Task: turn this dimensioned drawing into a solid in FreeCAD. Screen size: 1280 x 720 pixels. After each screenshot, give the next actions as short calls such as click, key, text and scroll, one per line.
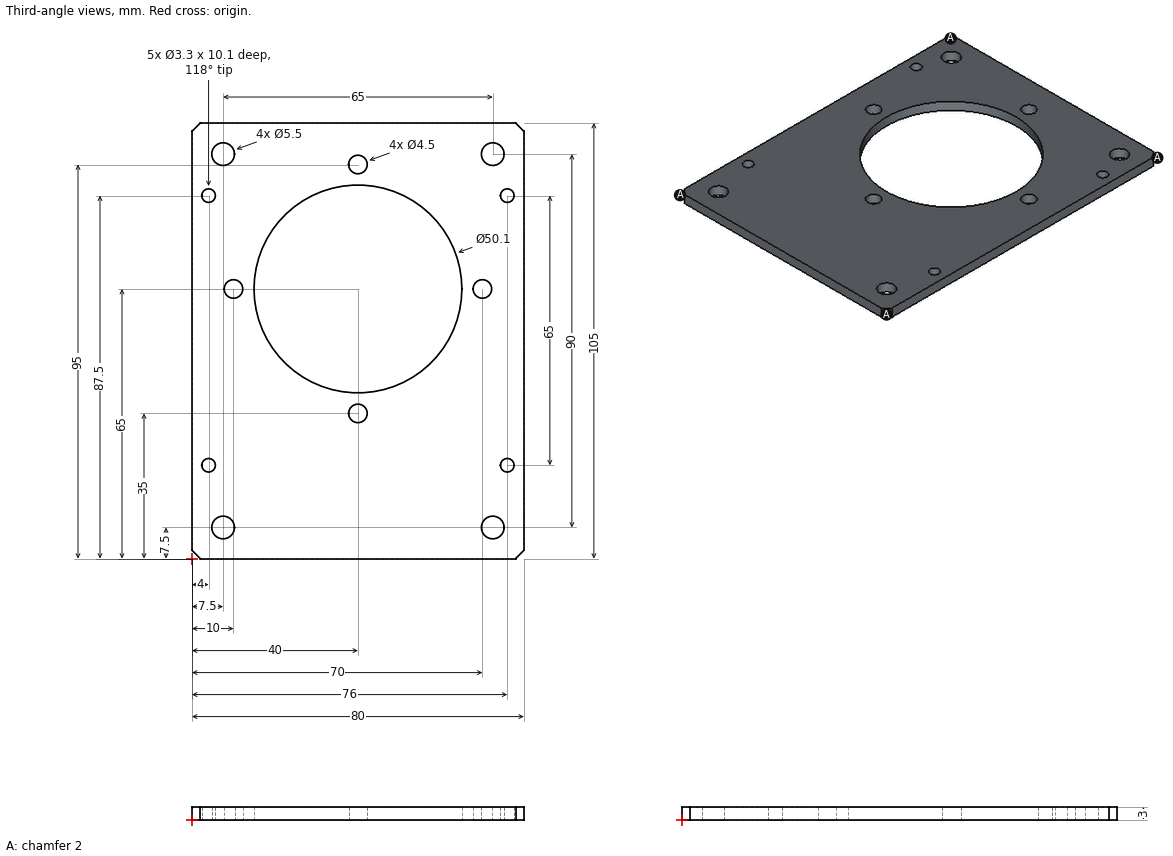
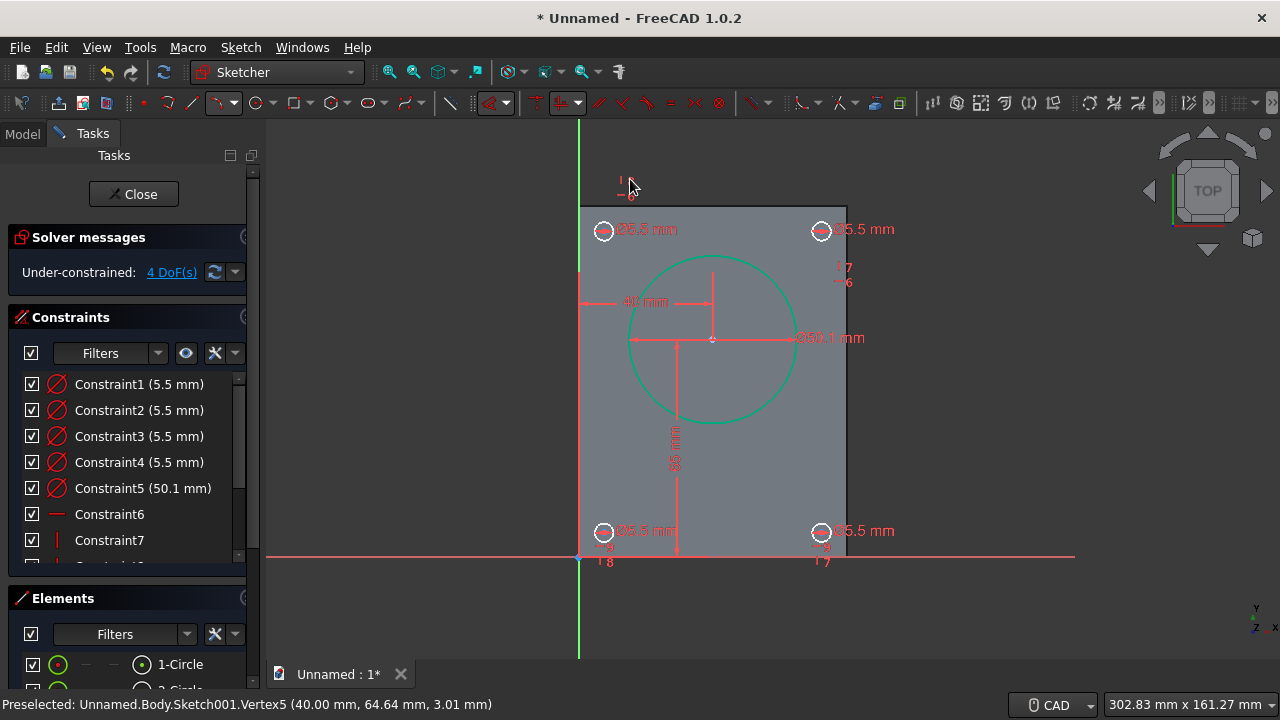
scroll(604, 231, up, 3)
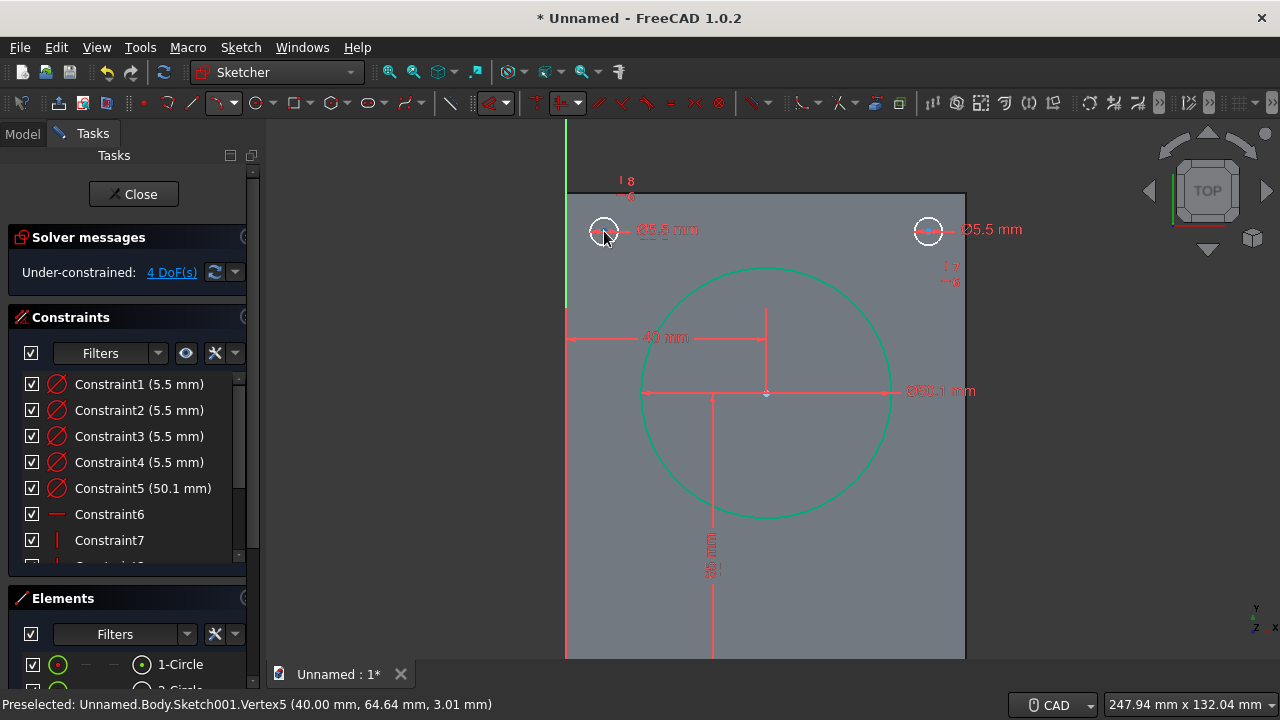
click(604, 232)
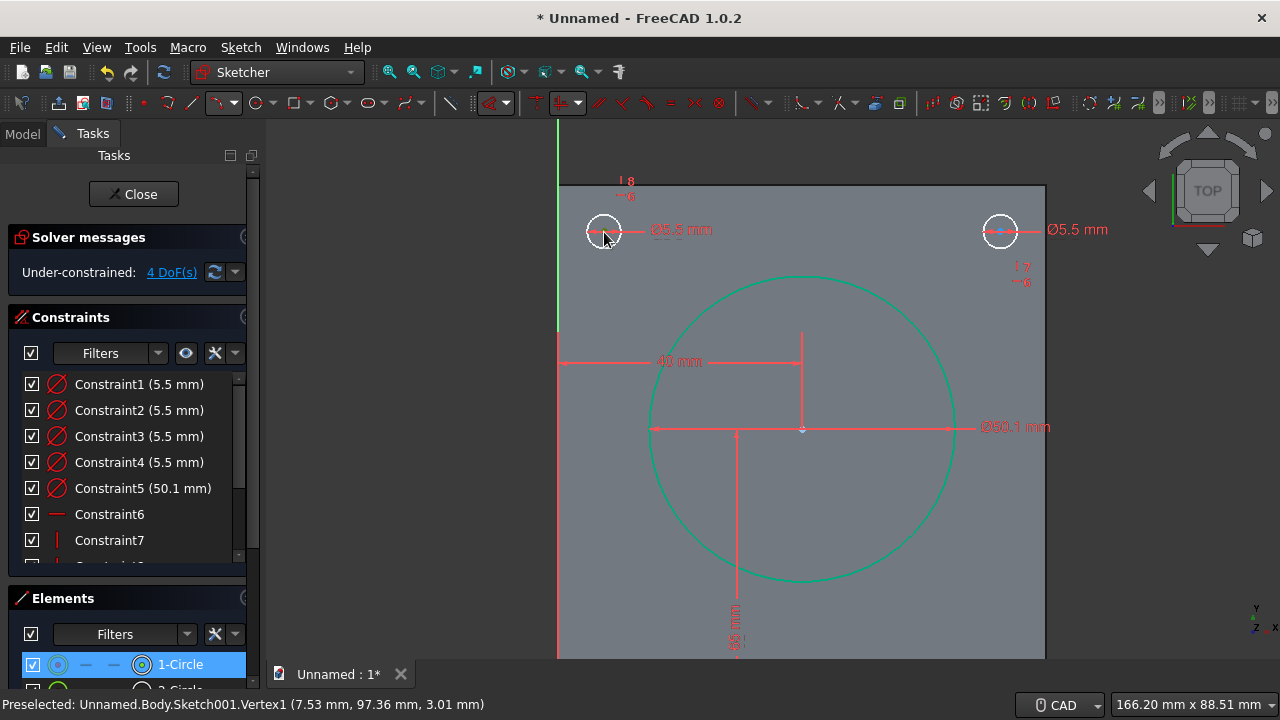
click(508, 104)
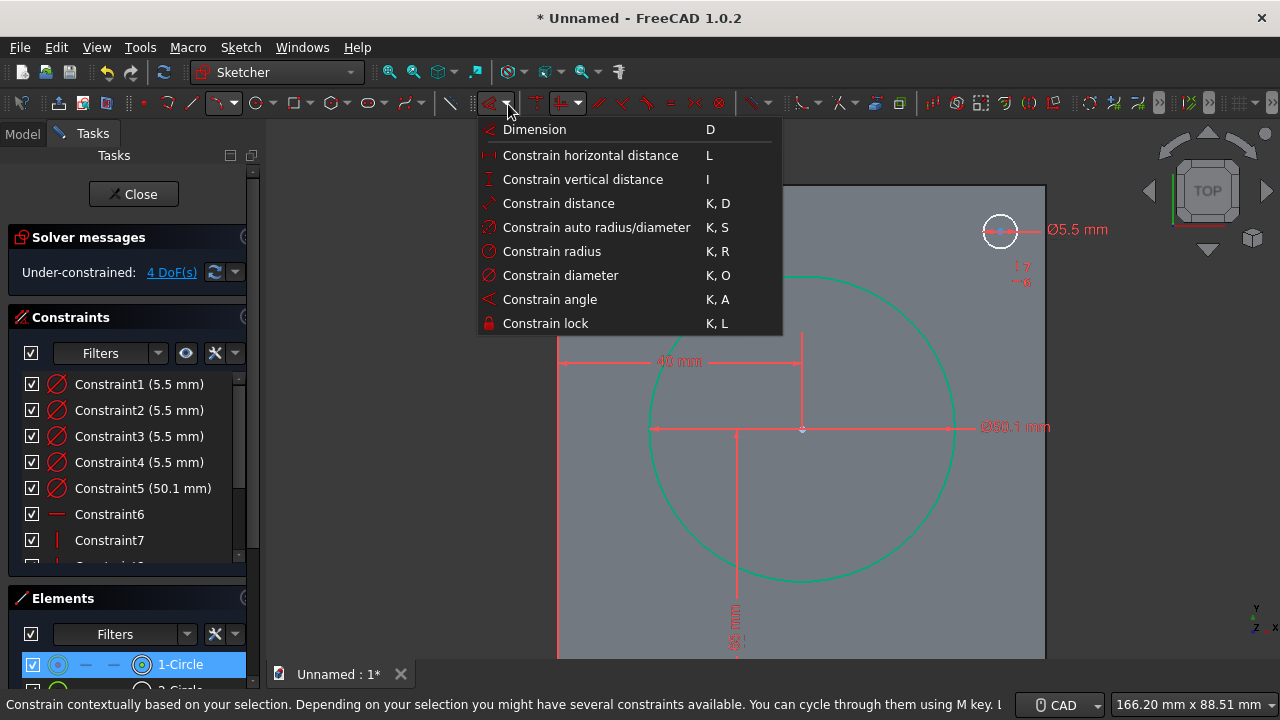
click(630, 155)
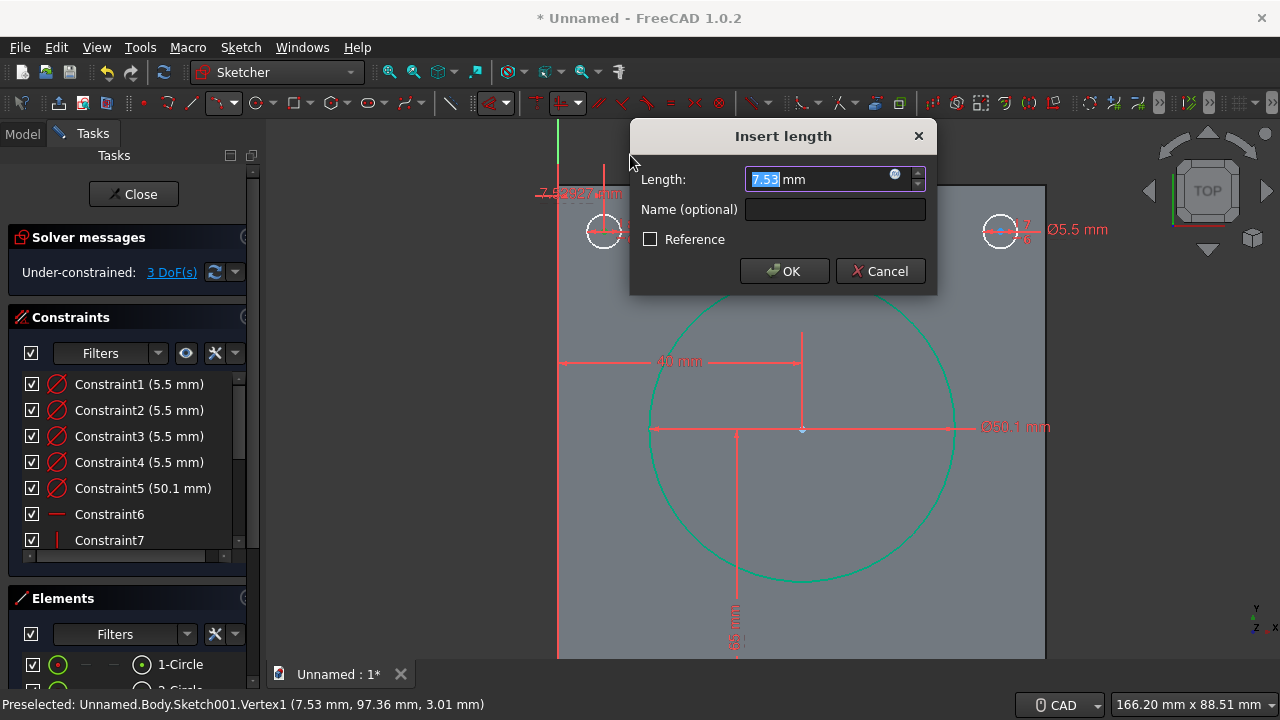
text(7.5)
key(Return)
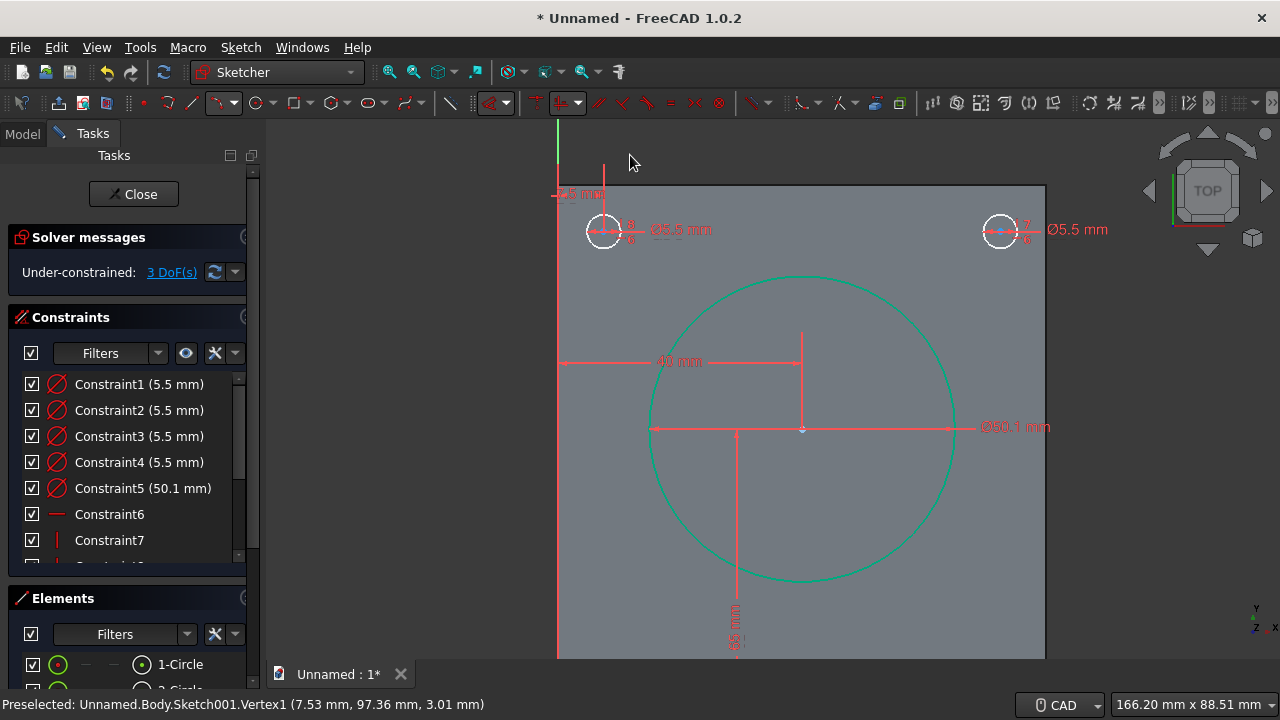
scroll(603, 230, down, 3)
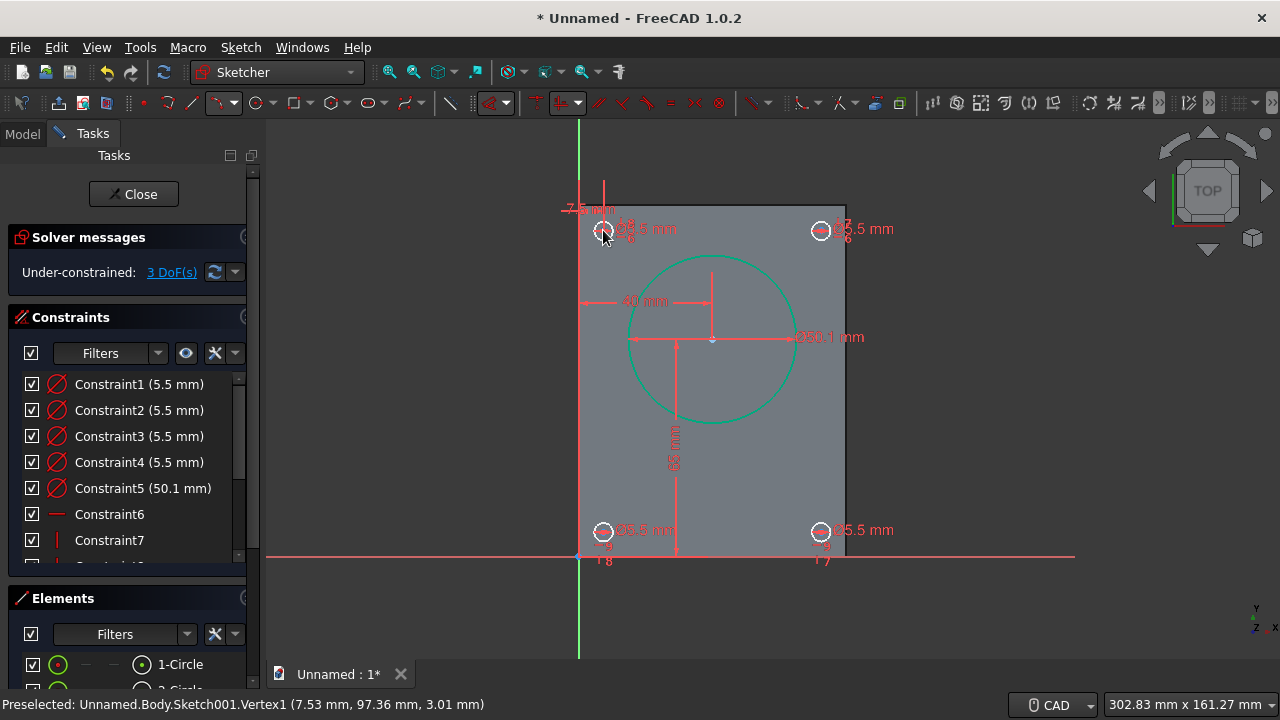
scroll(821, 532, up, 3)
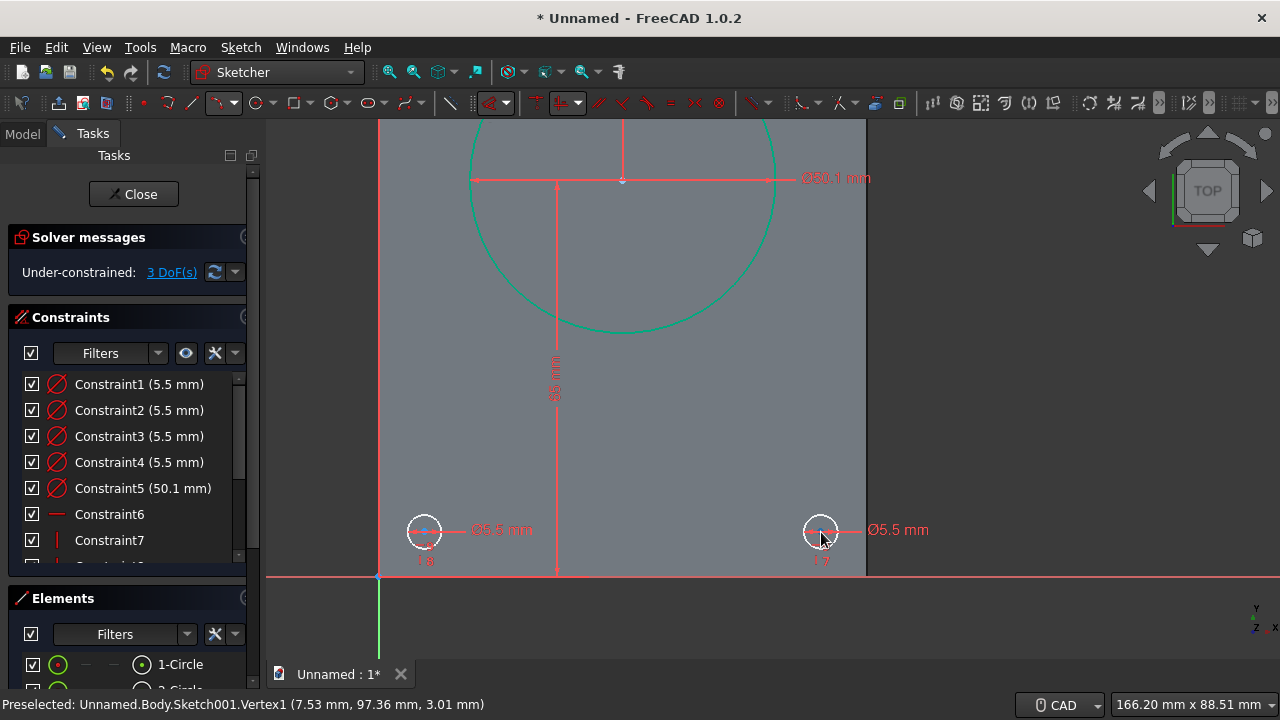
click(821, 532)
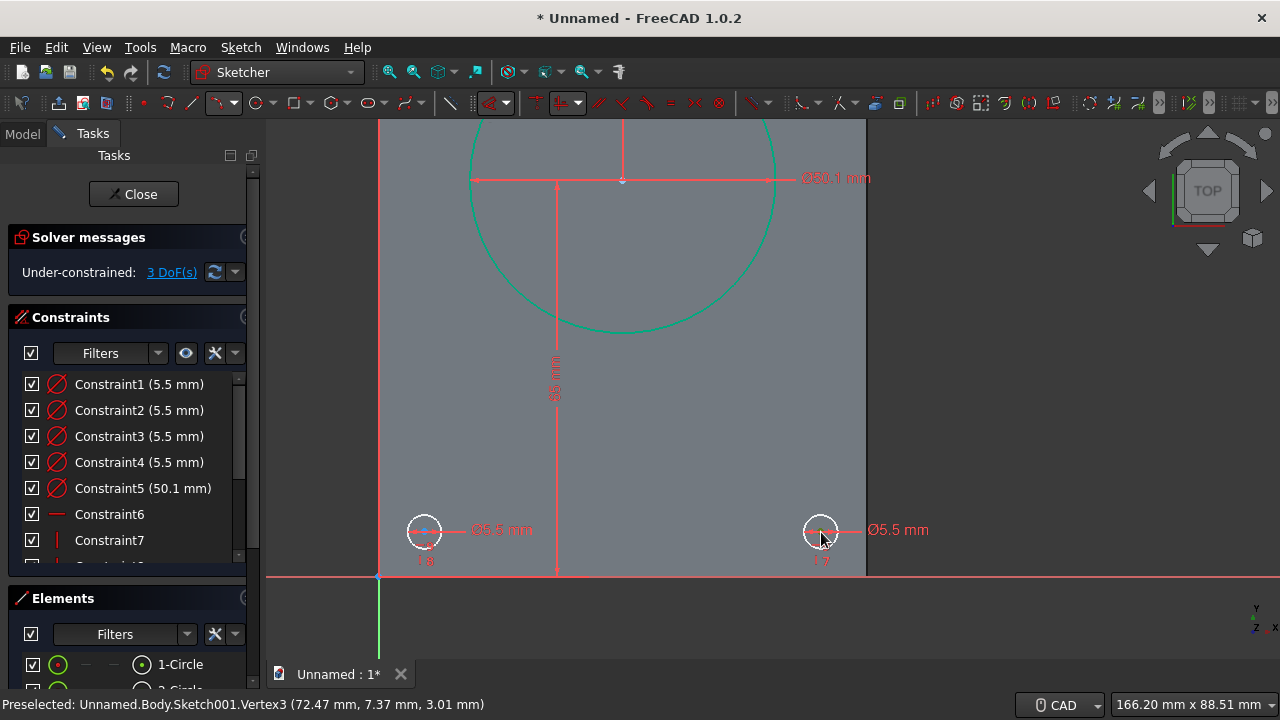
click(508, 104)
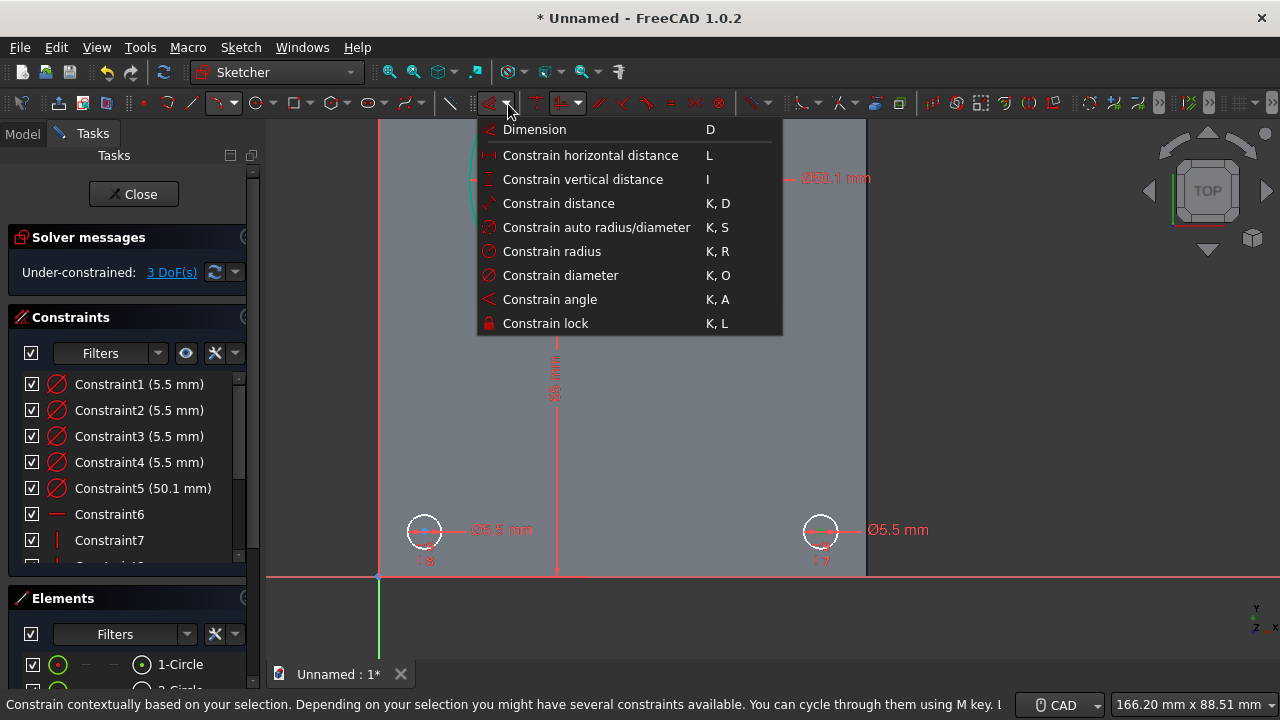
click(630, 179)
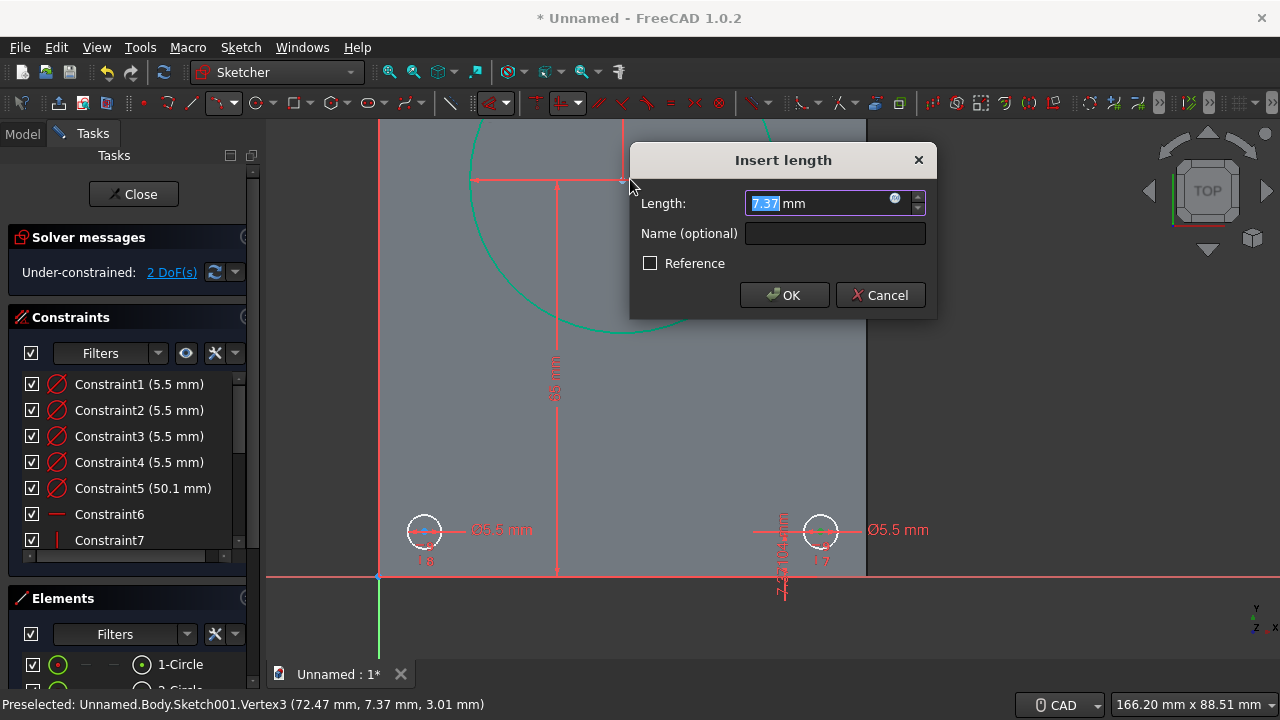
text(7.5)
key(Return)